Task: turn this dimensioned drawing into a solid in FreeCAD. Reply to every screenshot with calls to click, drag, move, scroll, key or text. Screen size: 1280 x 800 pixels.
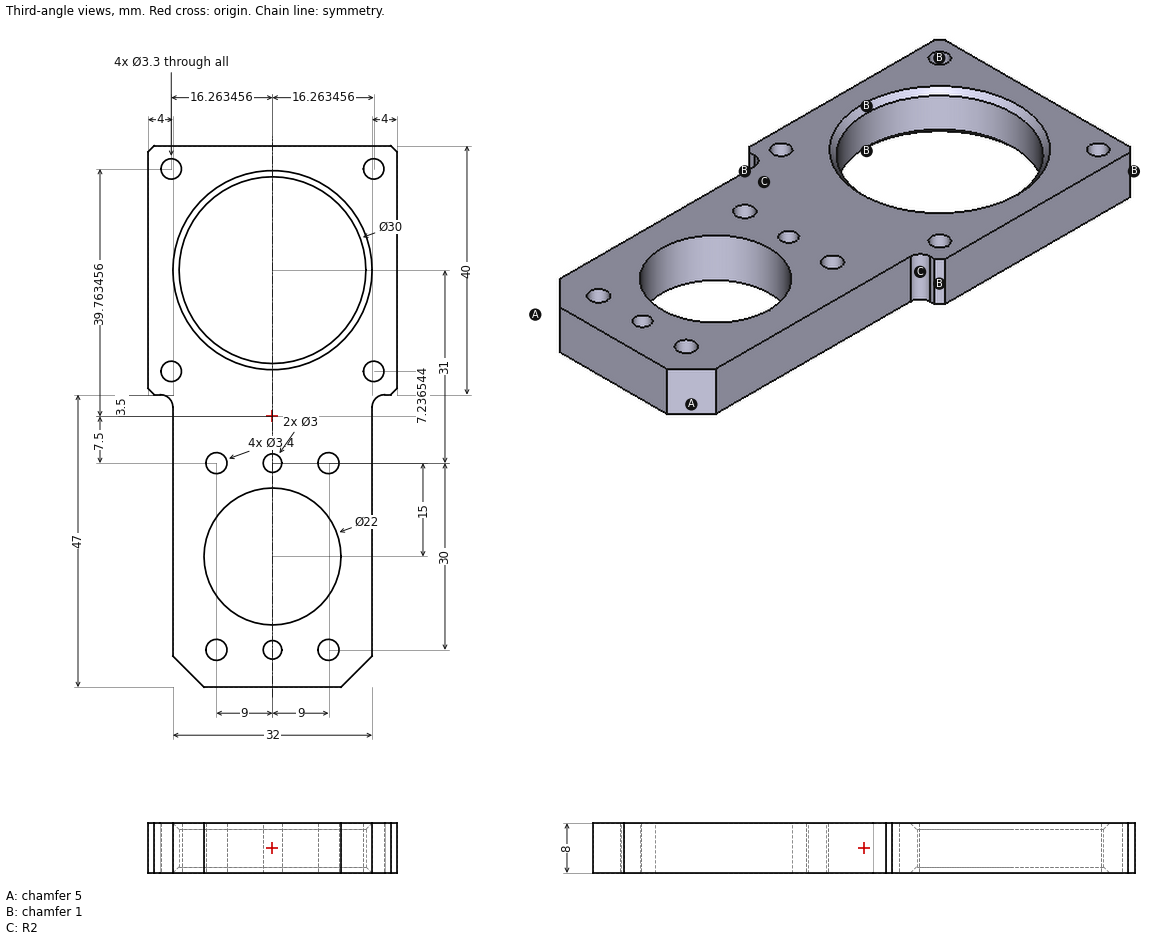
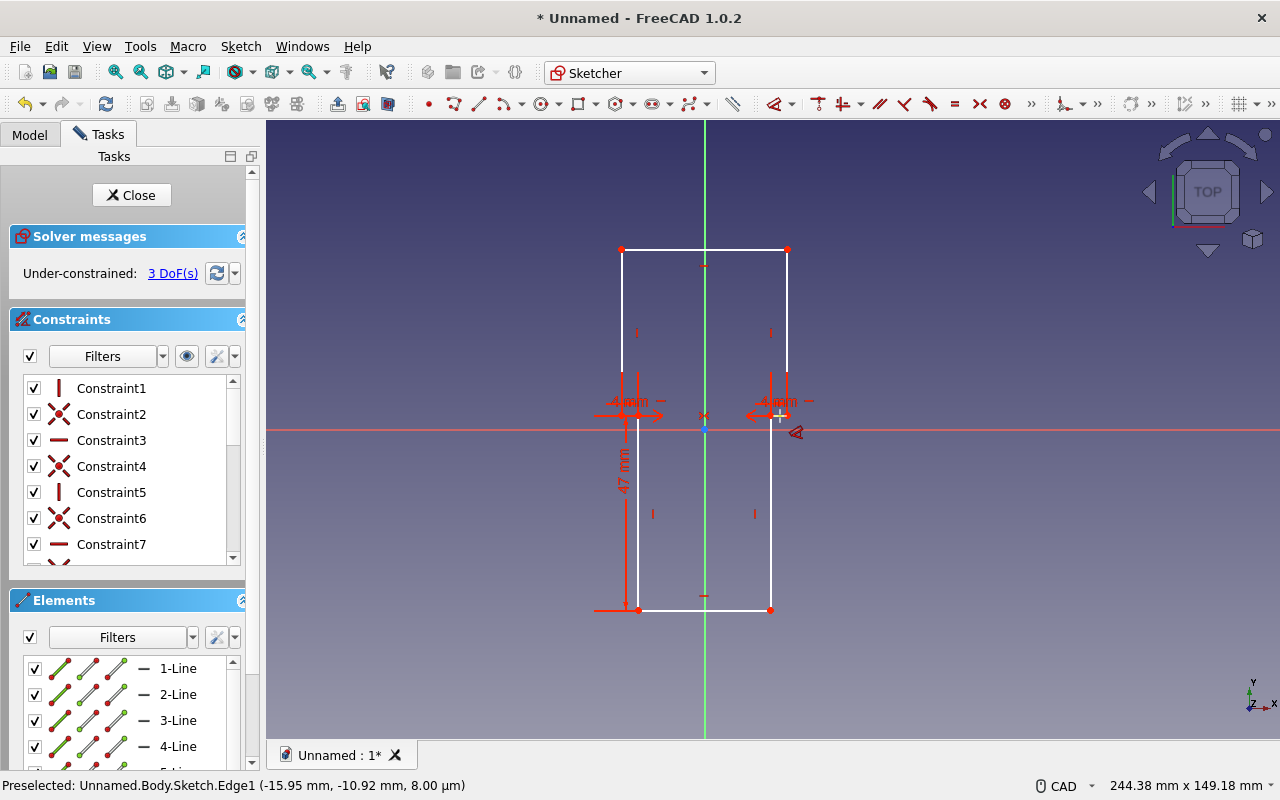
click(678, 611)
click(674, 645)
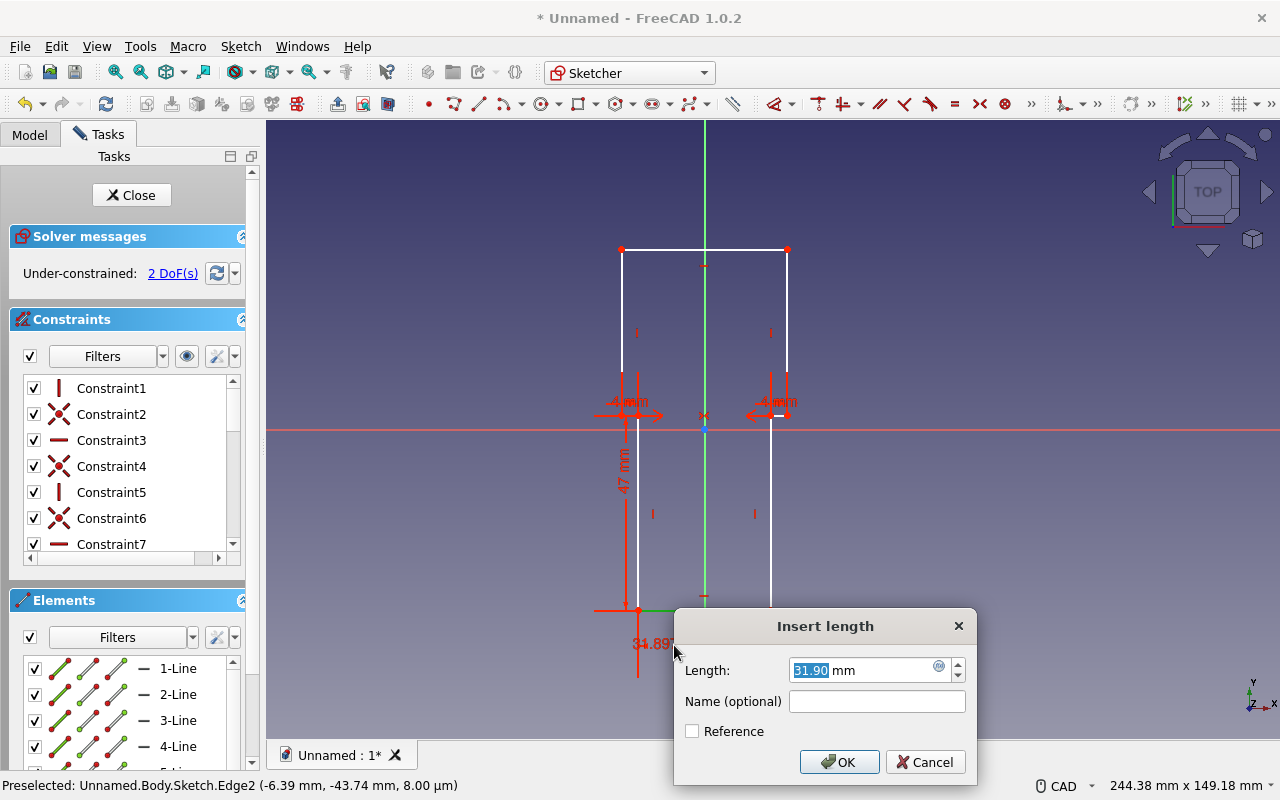
text(32)
key(Return)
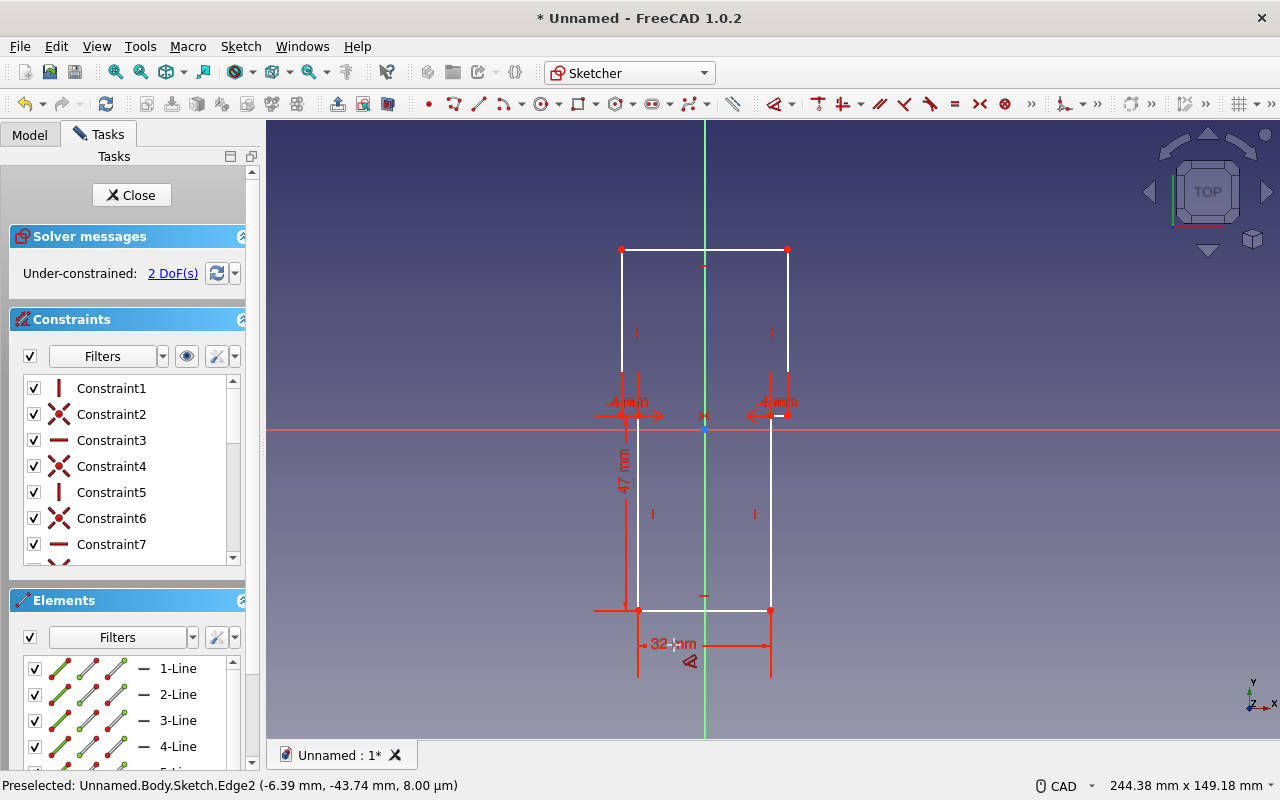
click(788, 366)
click(822, 333)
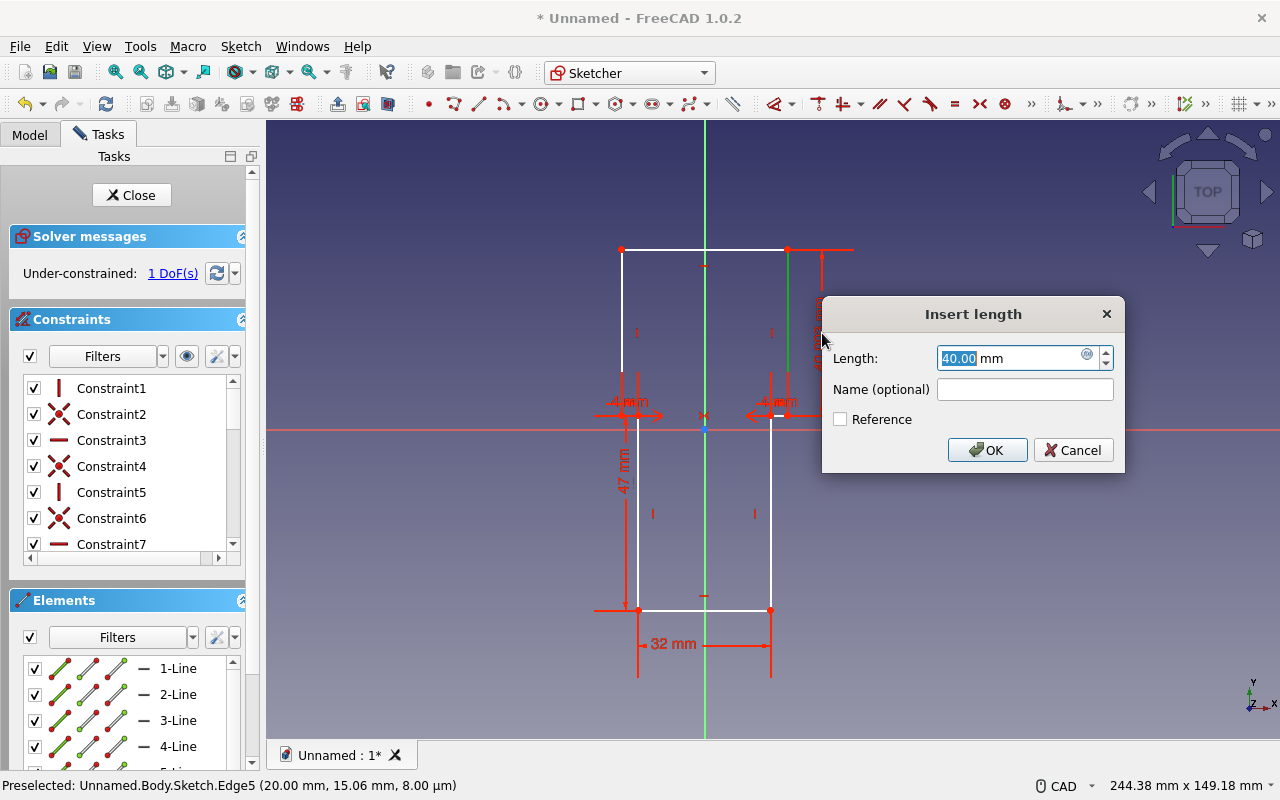
text(40)
key(Return)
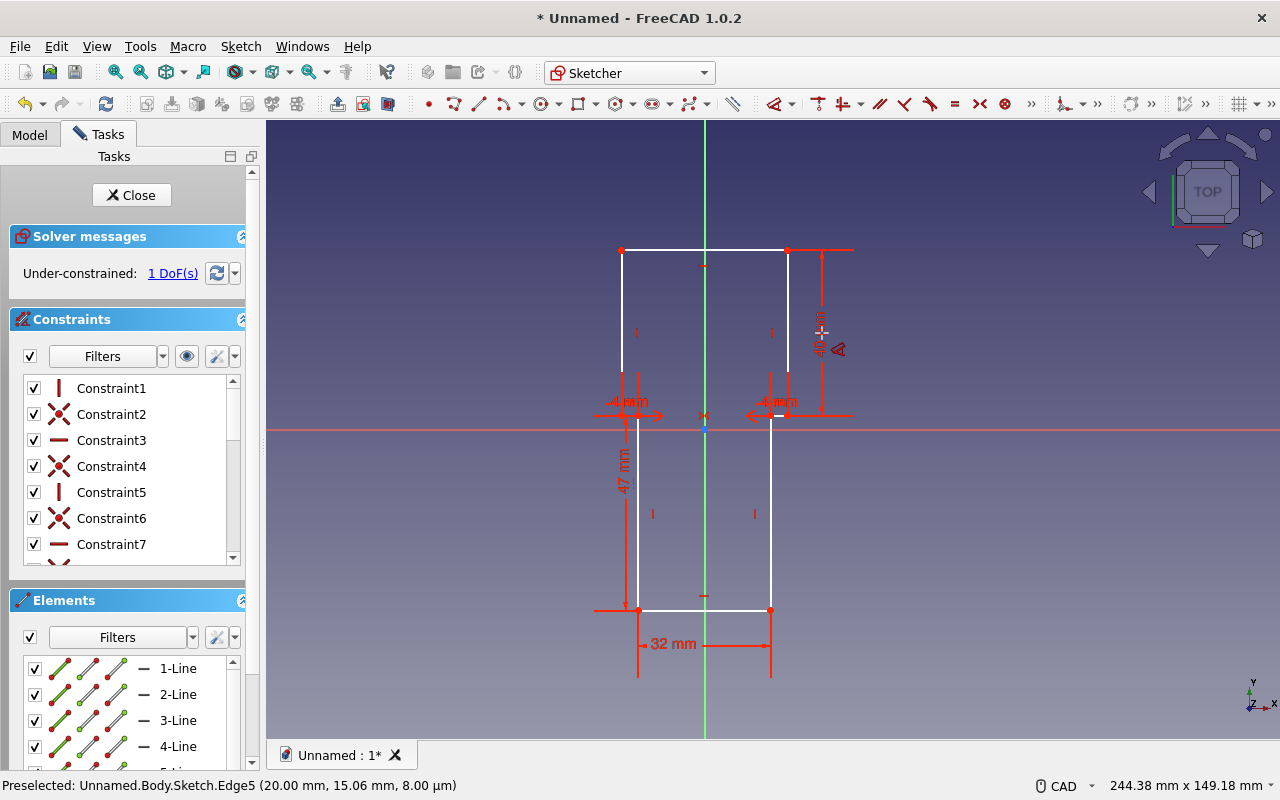
scroll(638, 416, up, 6)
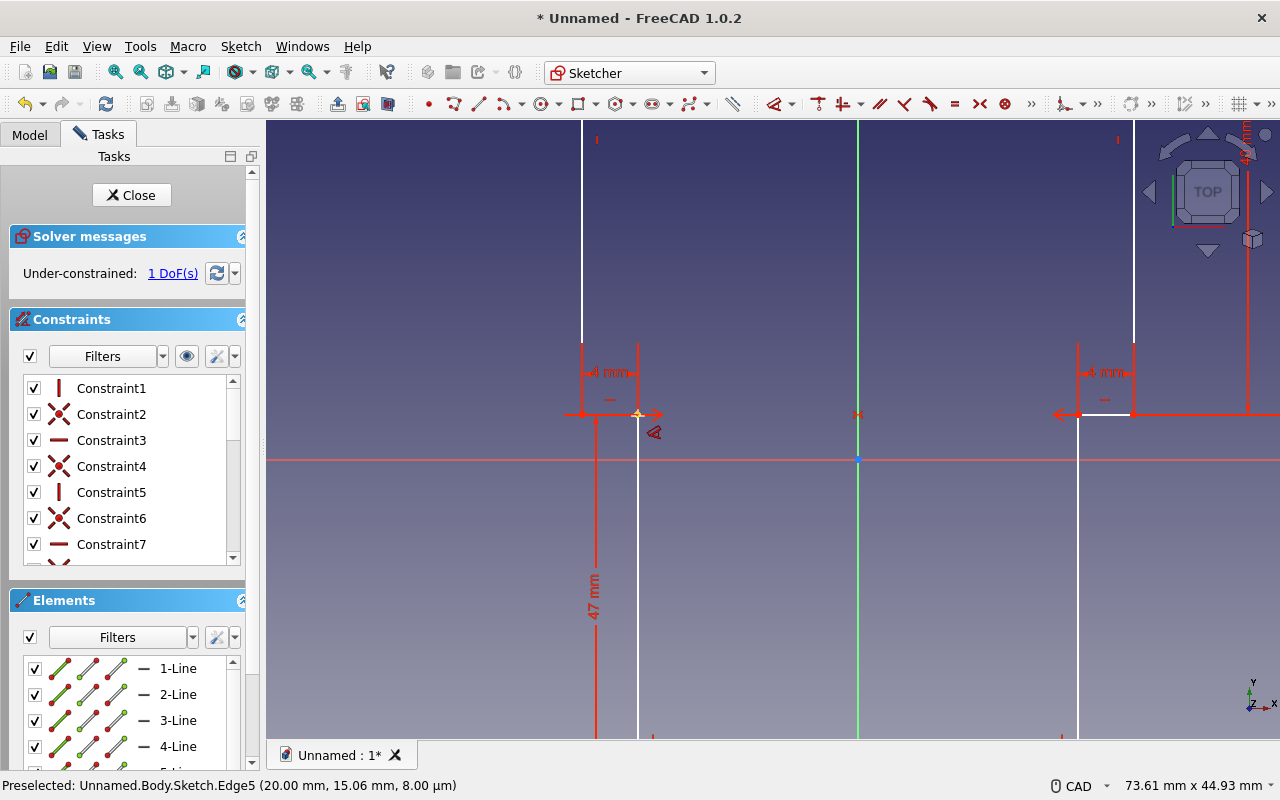
click(638, 415)
click(604, 437)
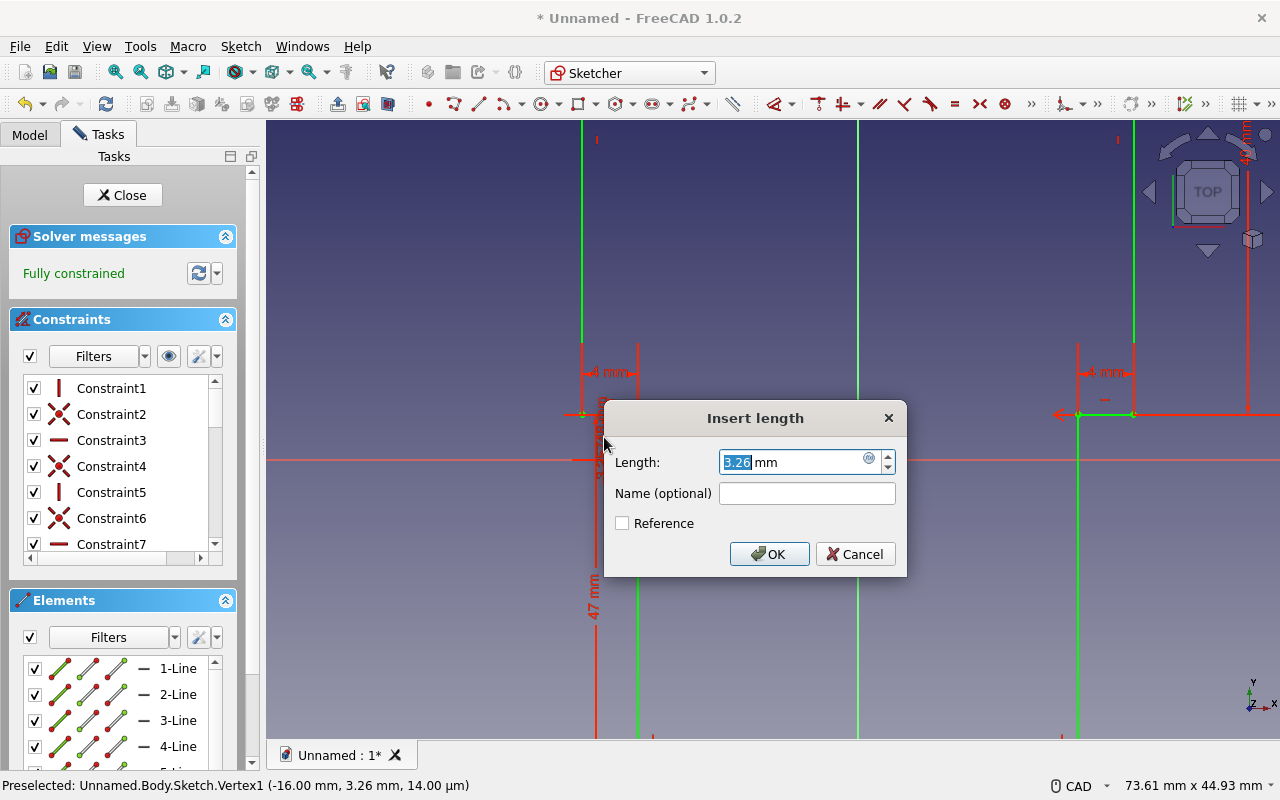
text(3.5)
key(Return)
key(Escape)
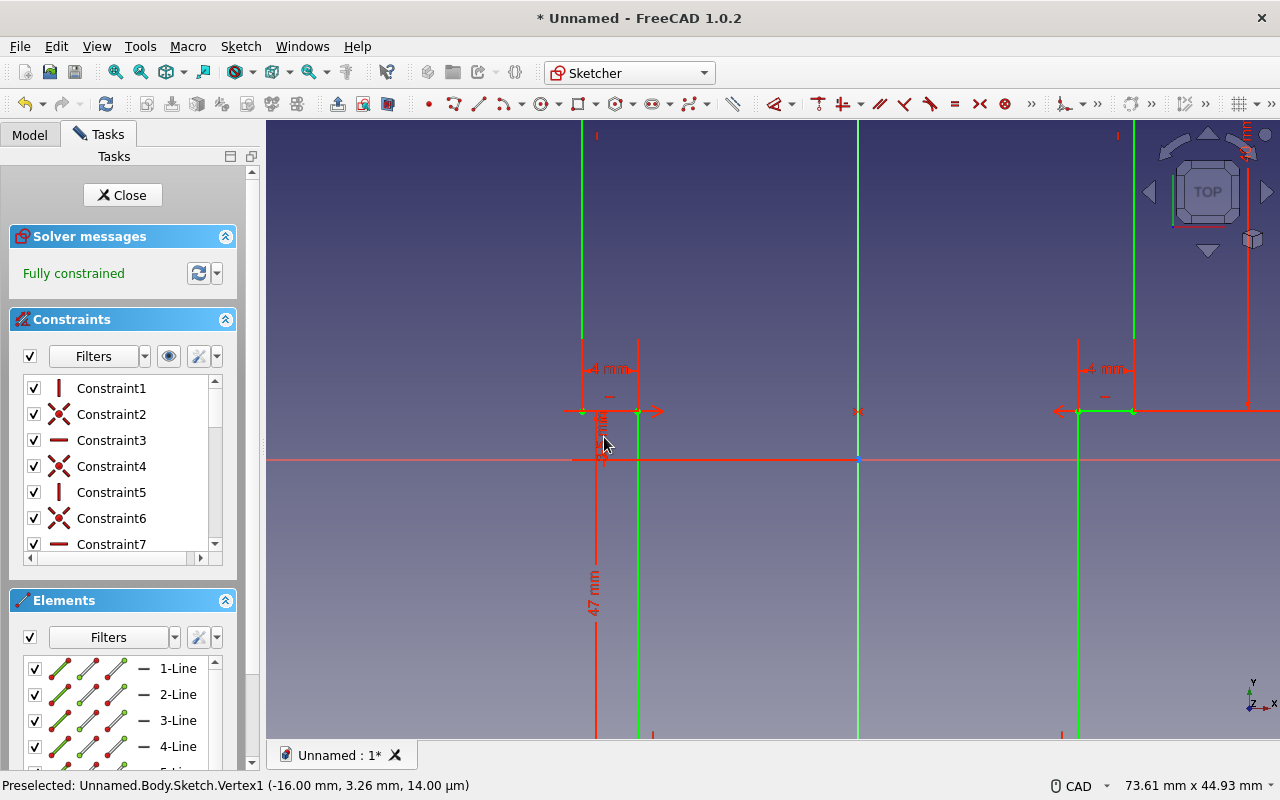
click(123, 195)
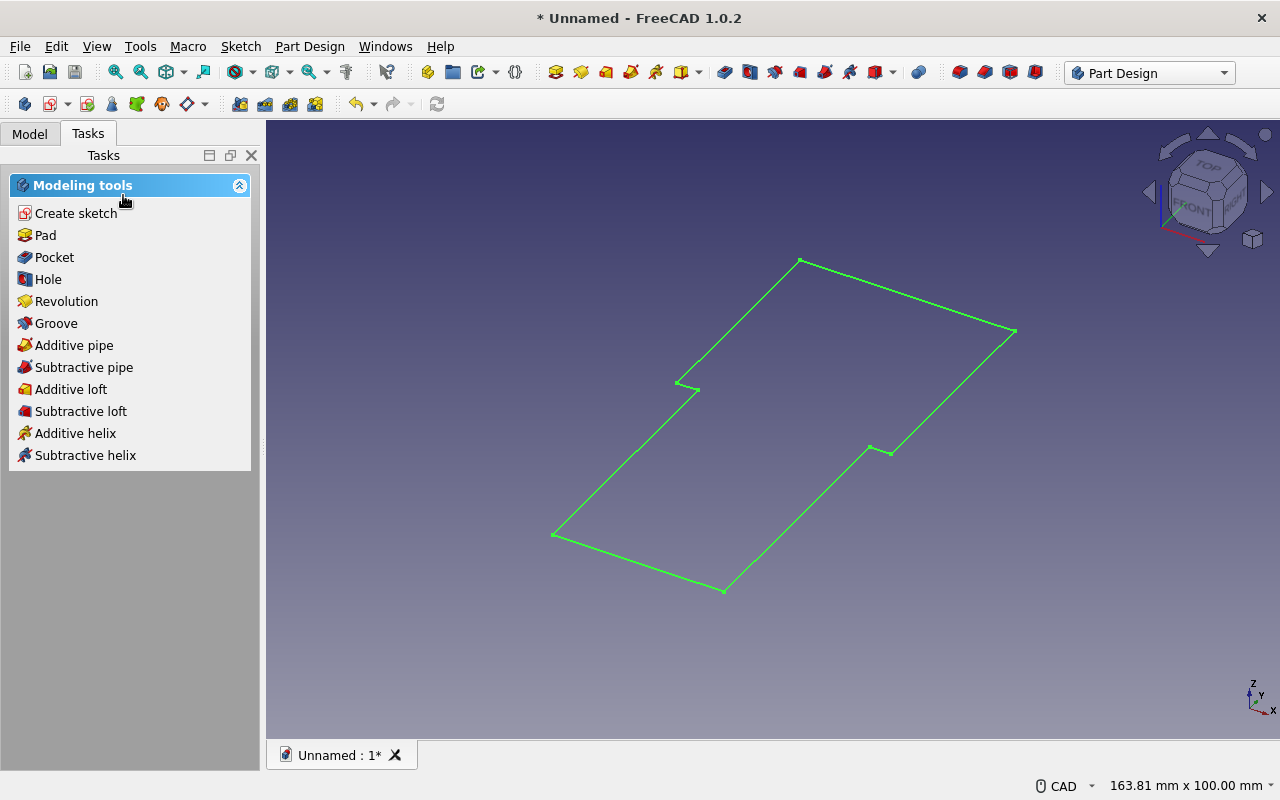
click(556, 72)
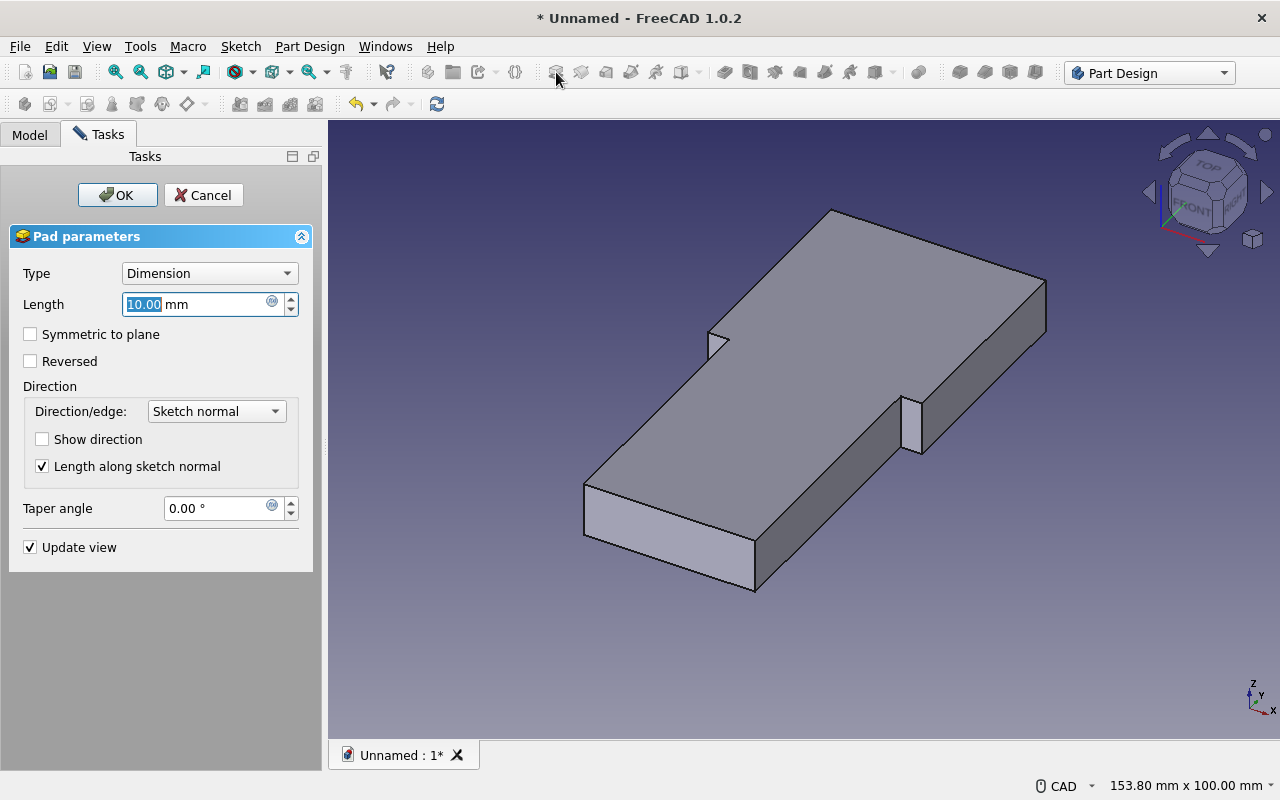
text(8)
key(Tab)